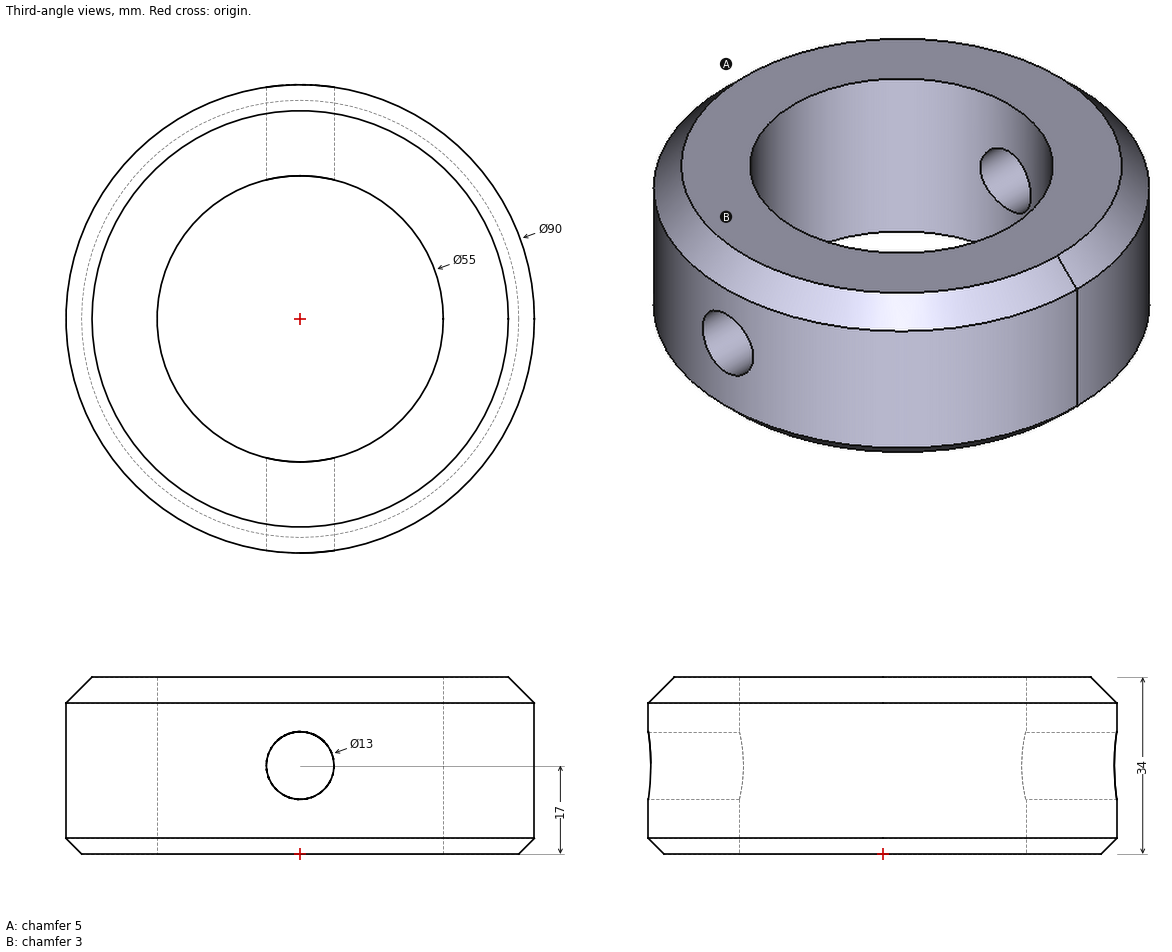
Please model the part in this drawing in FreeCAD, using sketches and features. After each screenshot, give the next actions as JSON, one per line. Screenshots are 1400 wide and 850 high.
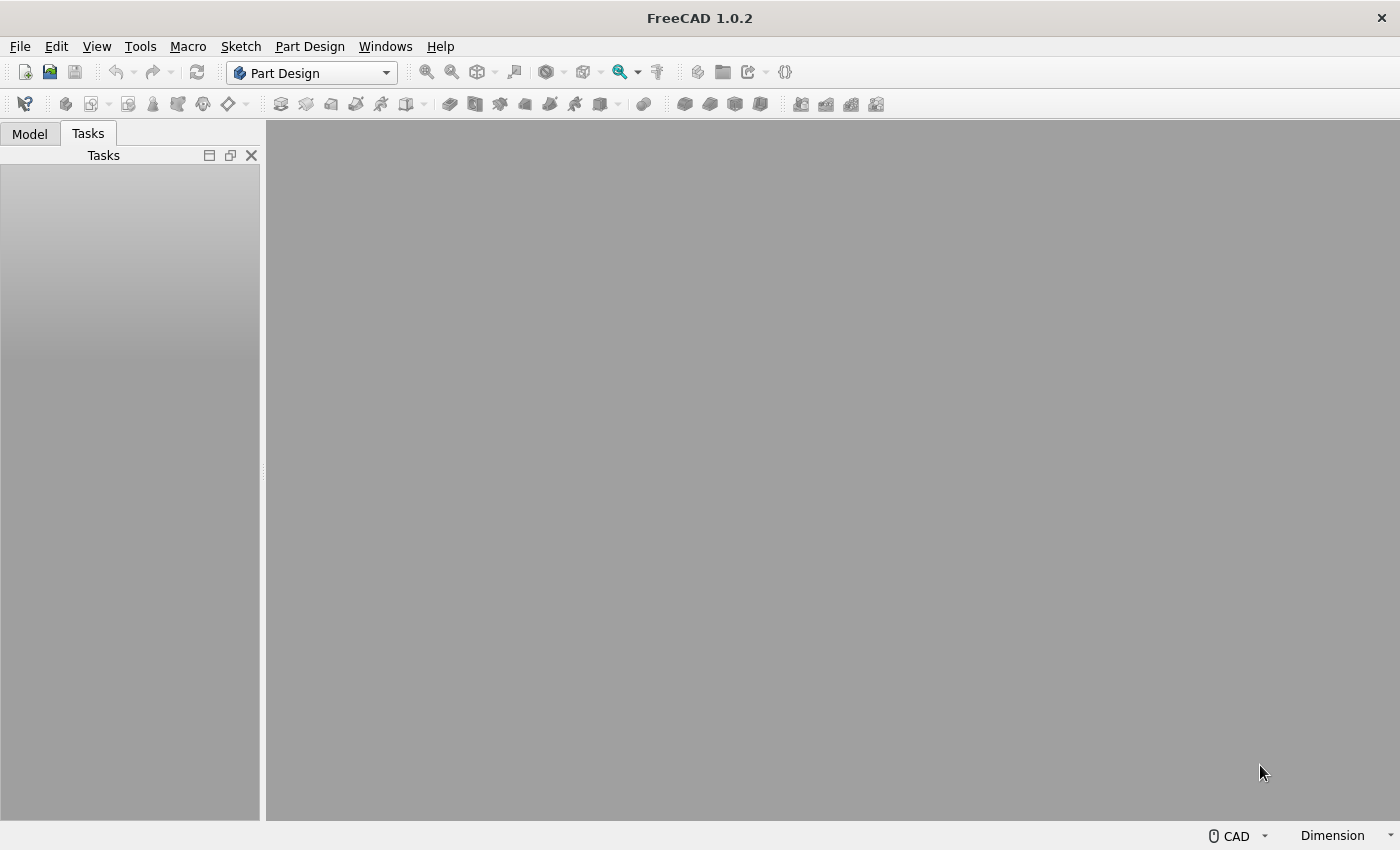
{"action": "key", "text": "ctrl+n"}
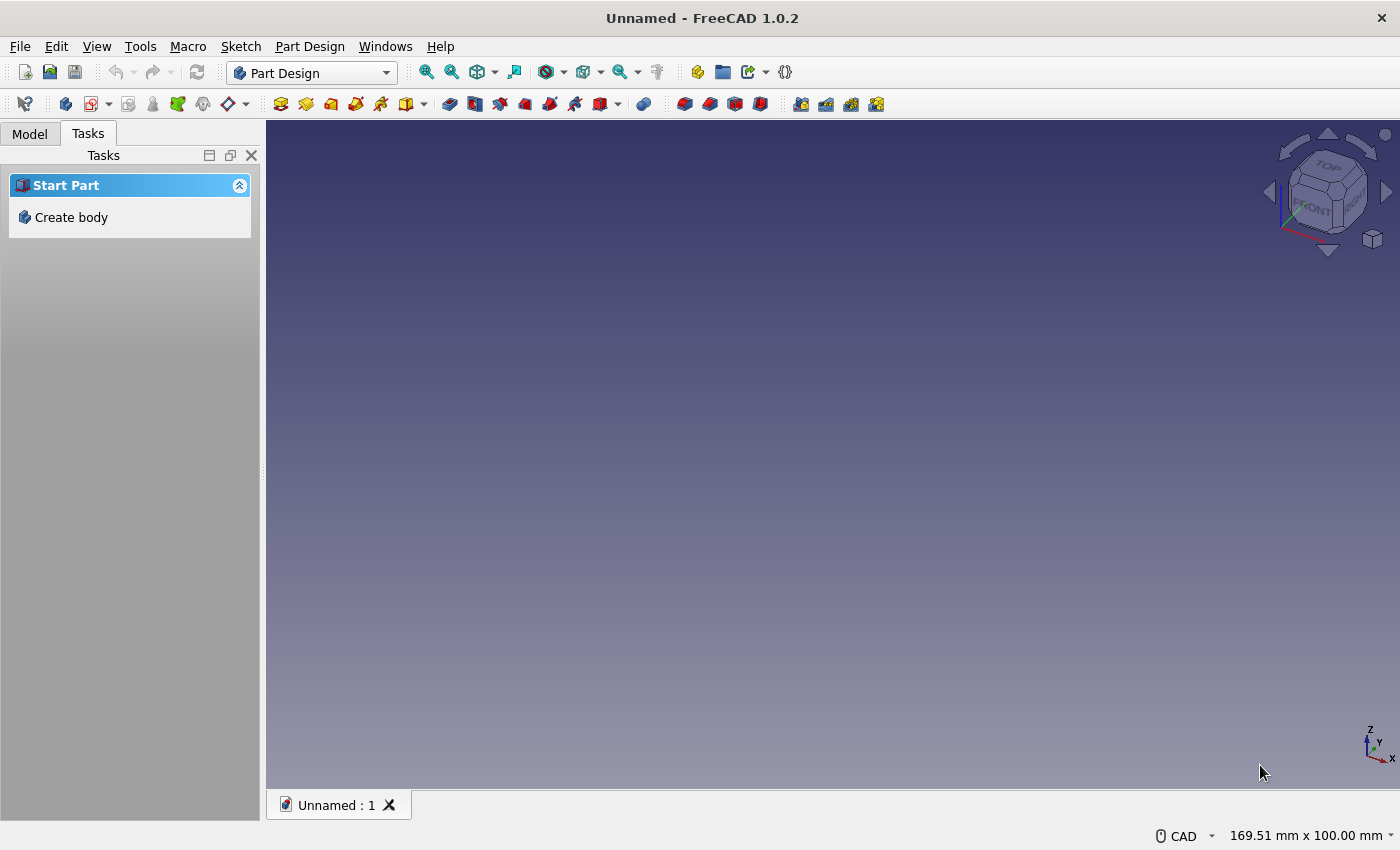
{"action": "left_click", "coordinate": [90, 104]}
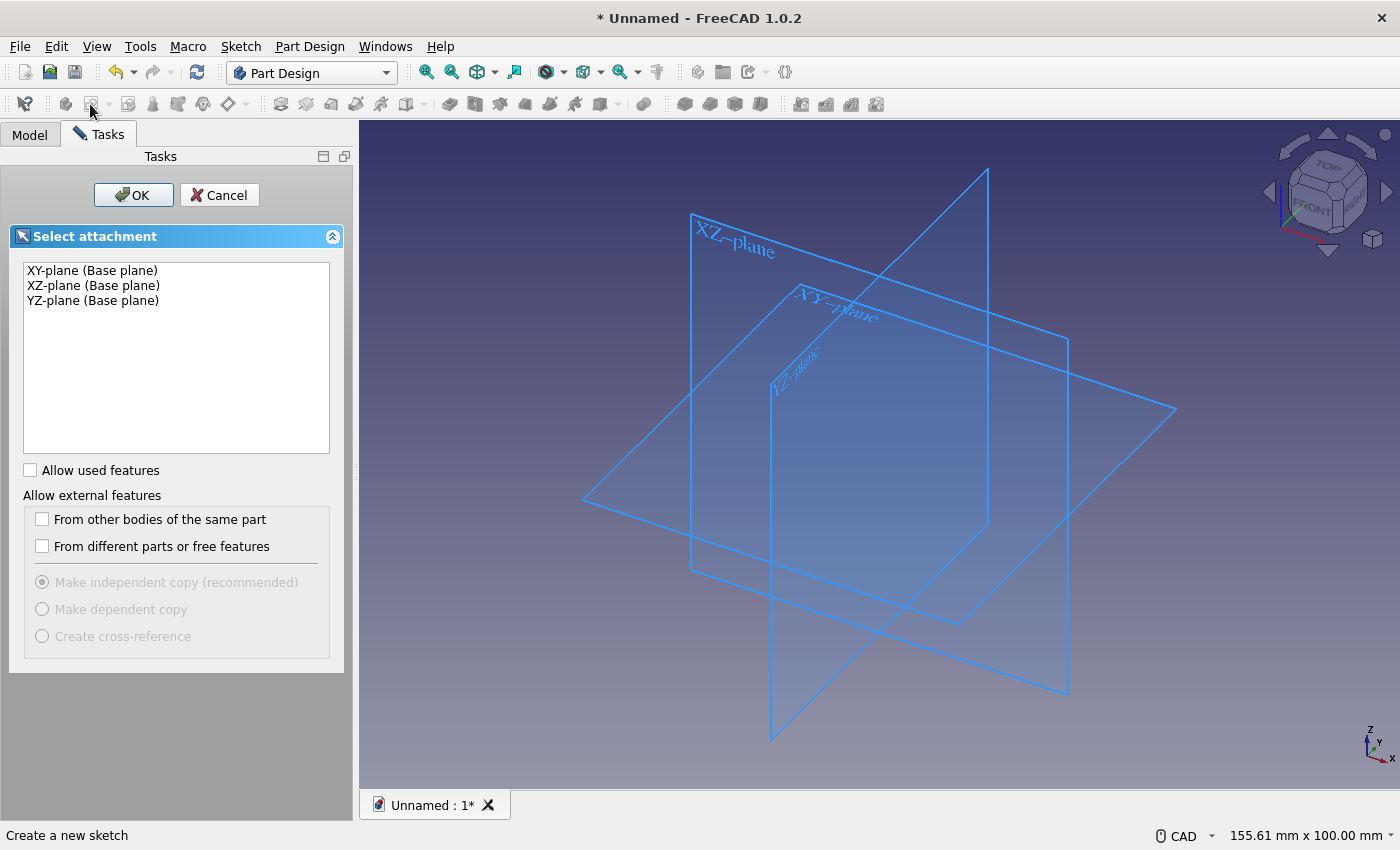
{"action": "left_click", "coordinate": [84, 270]}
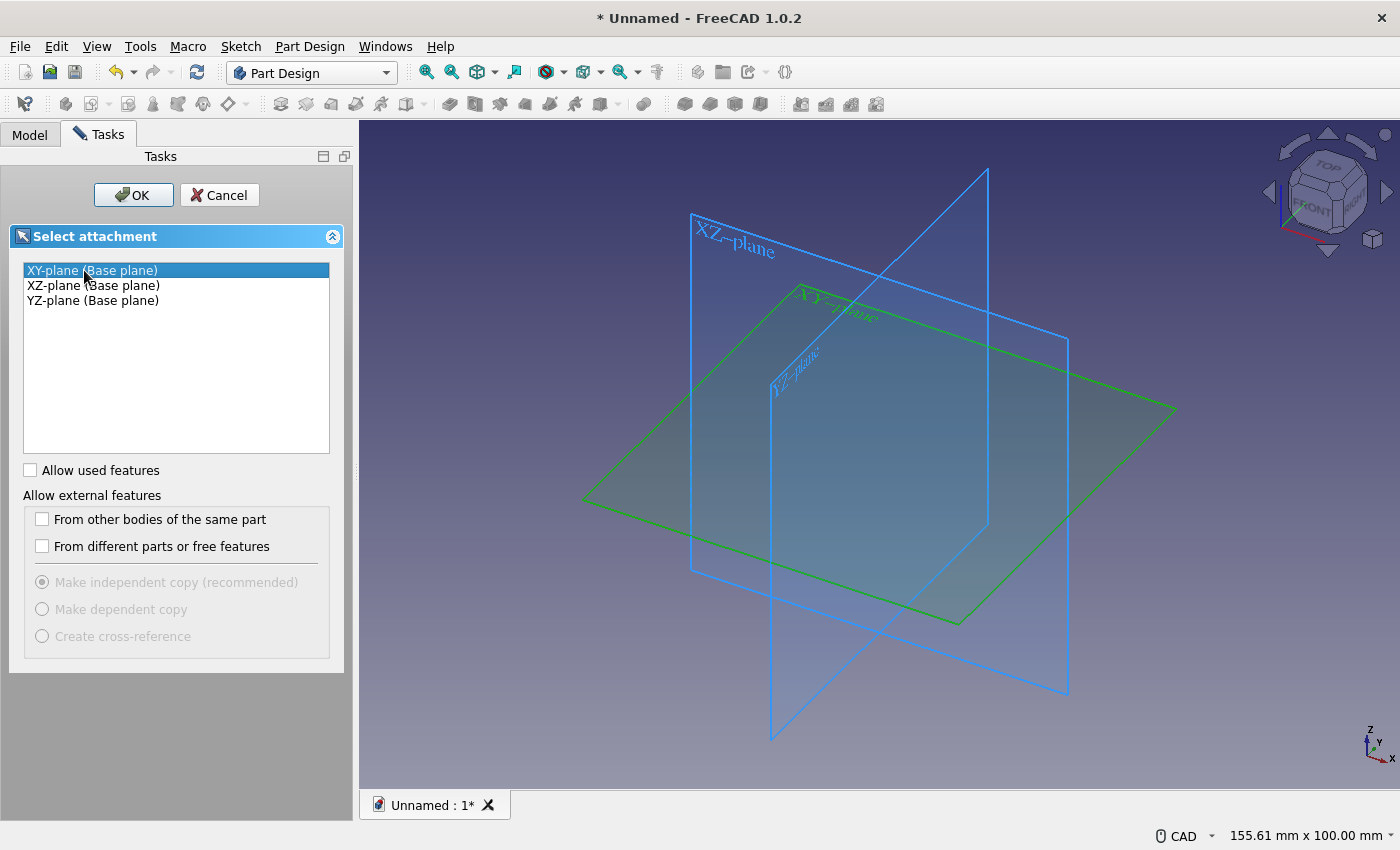
{"action": "left_click", "coordinate": [134, 195]}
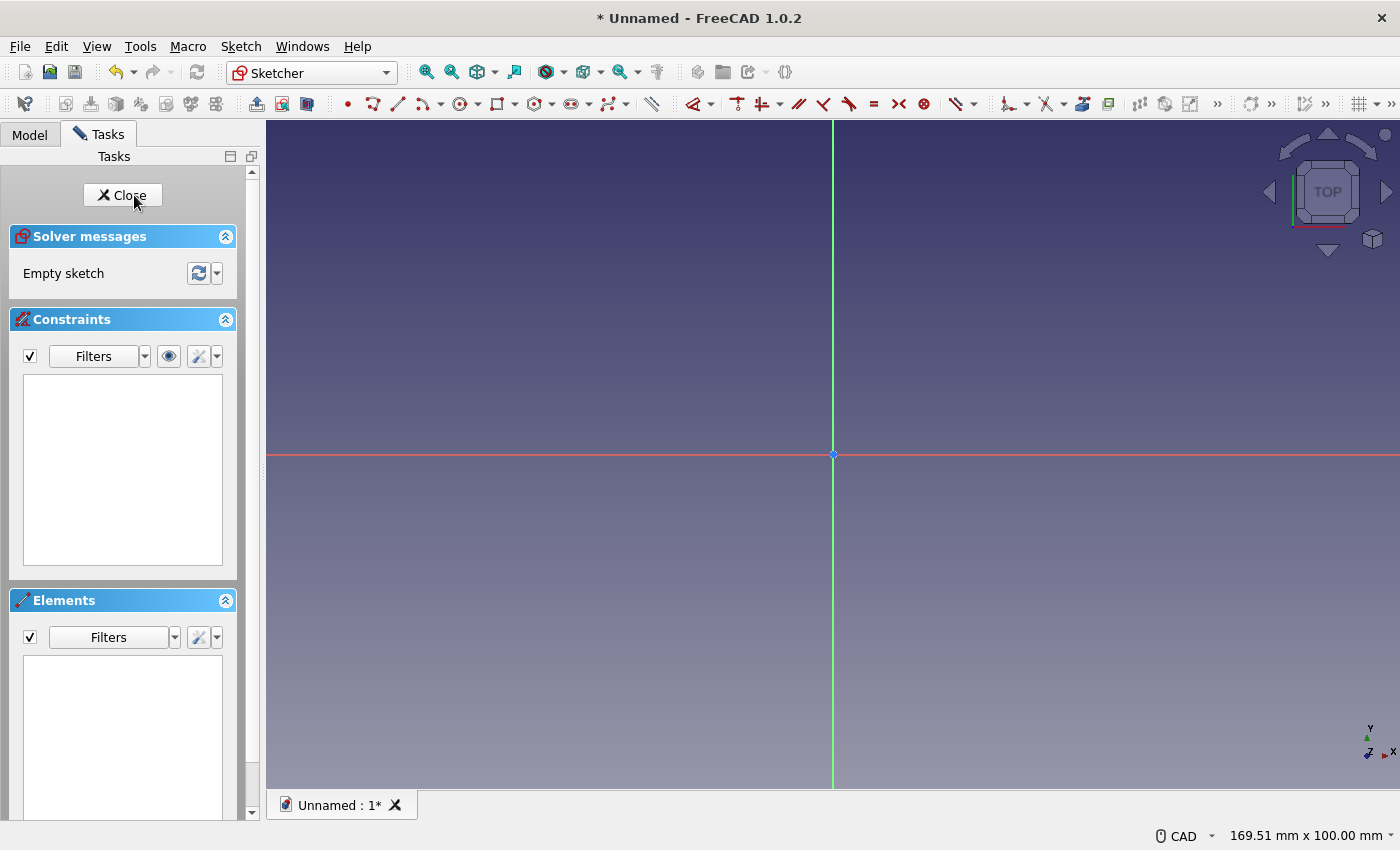
{"action": "scroll", "coordinate": [625, 455], "scroll_direction": "down", "scroll_amount": 2}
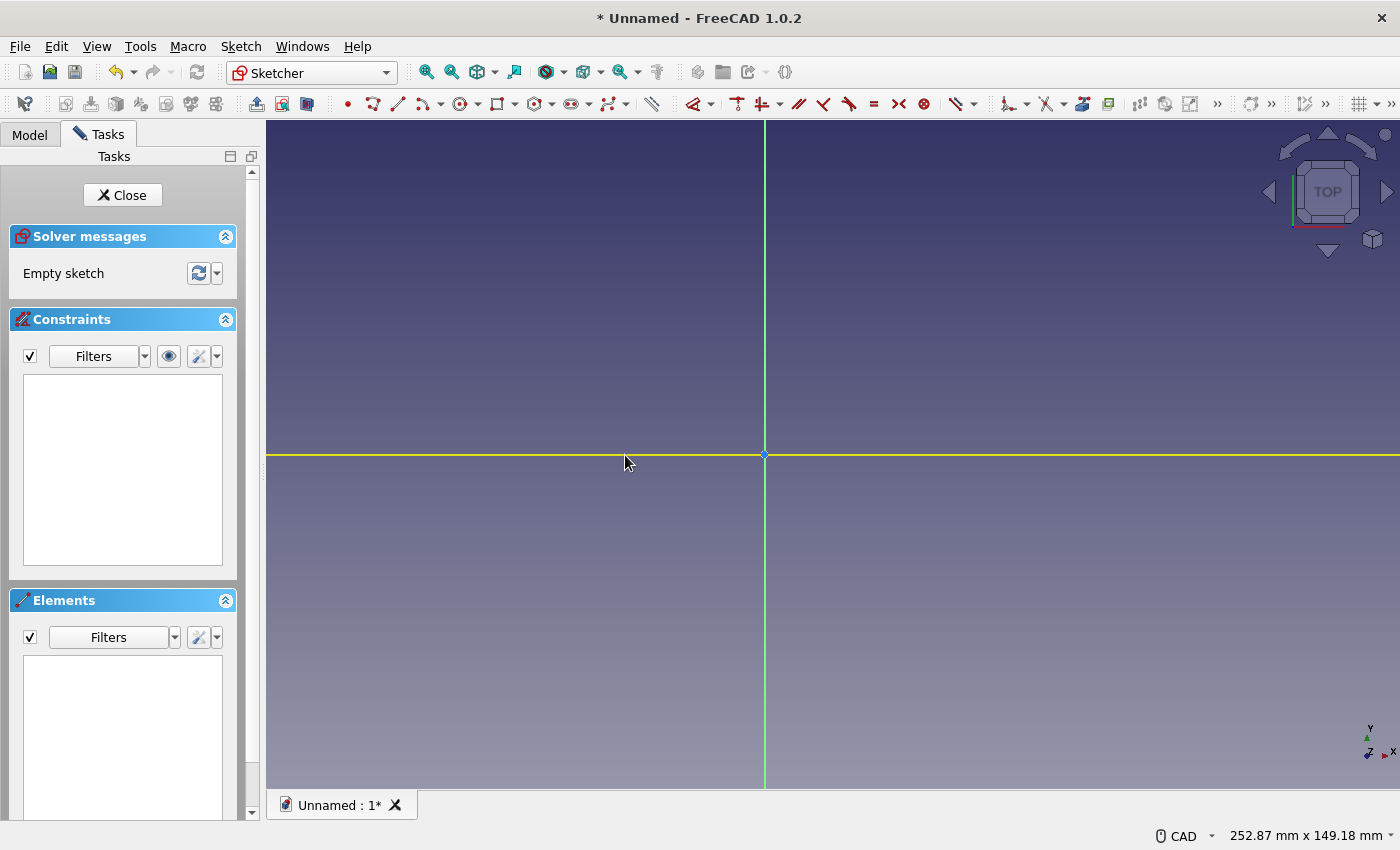
{"action": "key", "text": "g c"}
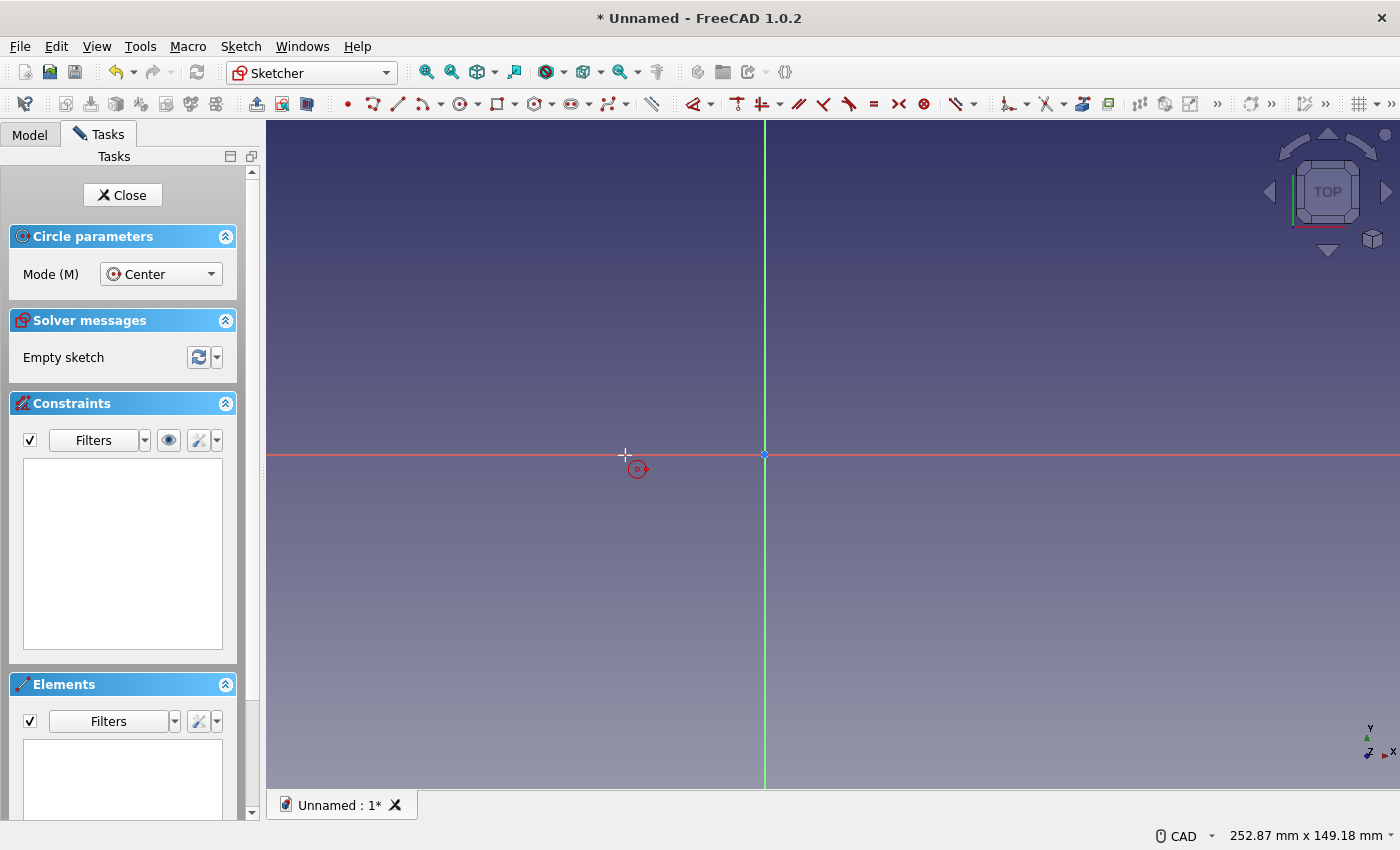
{"action": "left_click", "coordinate": [765, 455]}
{"action": "left_click", "coordinate": [907, 312]}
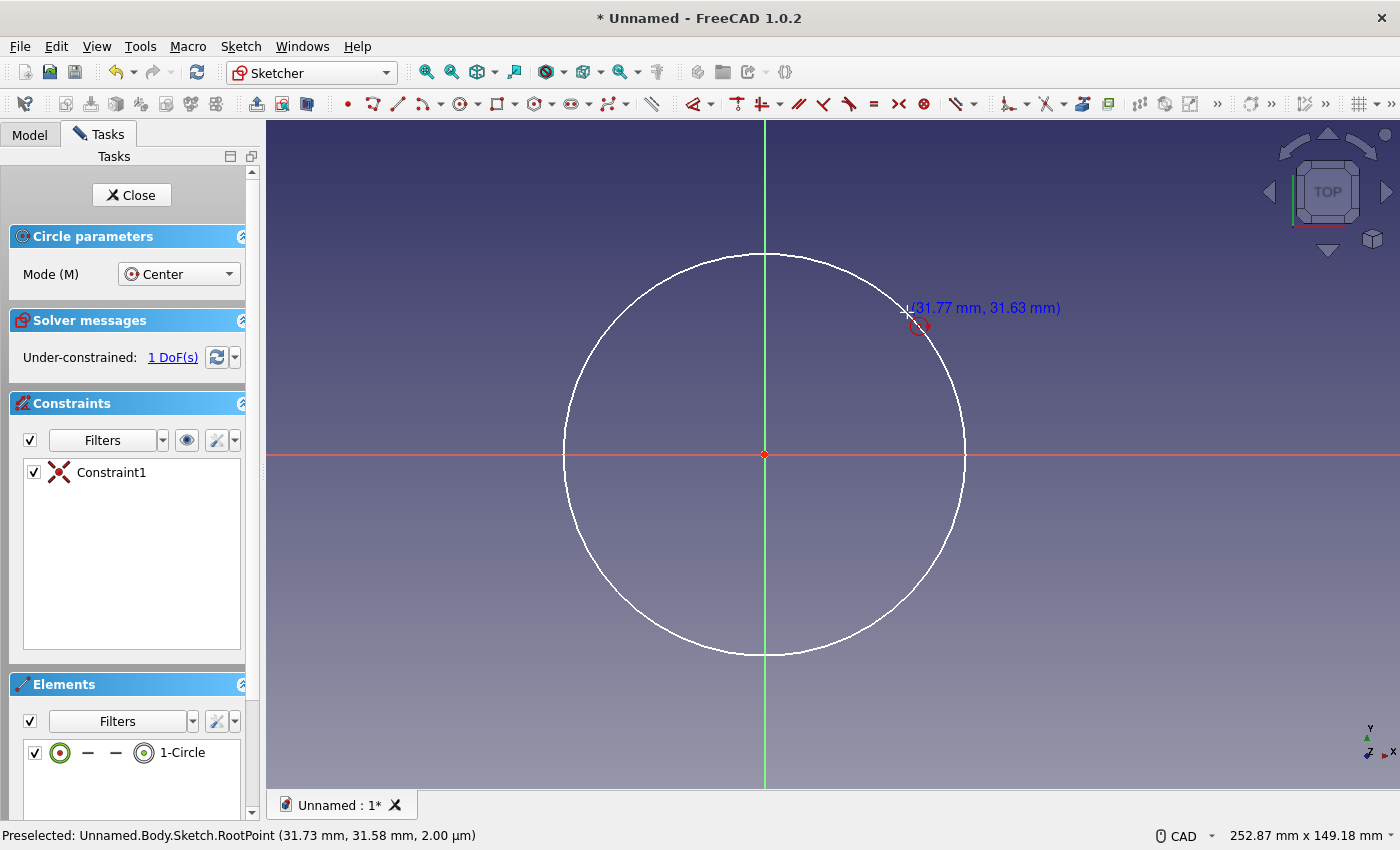
{"action": "left_click", "coordinate": [765, 455]}
{"action": "left_click", "coordinate": [852, 368]}
{"action": "key", "text": "Escape"}